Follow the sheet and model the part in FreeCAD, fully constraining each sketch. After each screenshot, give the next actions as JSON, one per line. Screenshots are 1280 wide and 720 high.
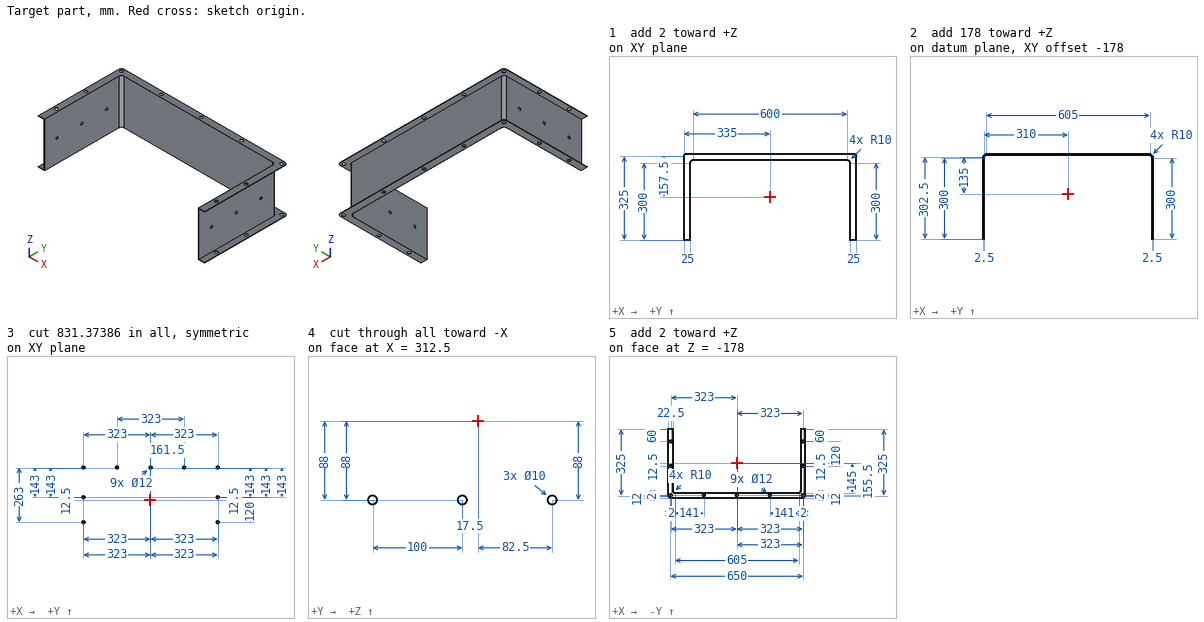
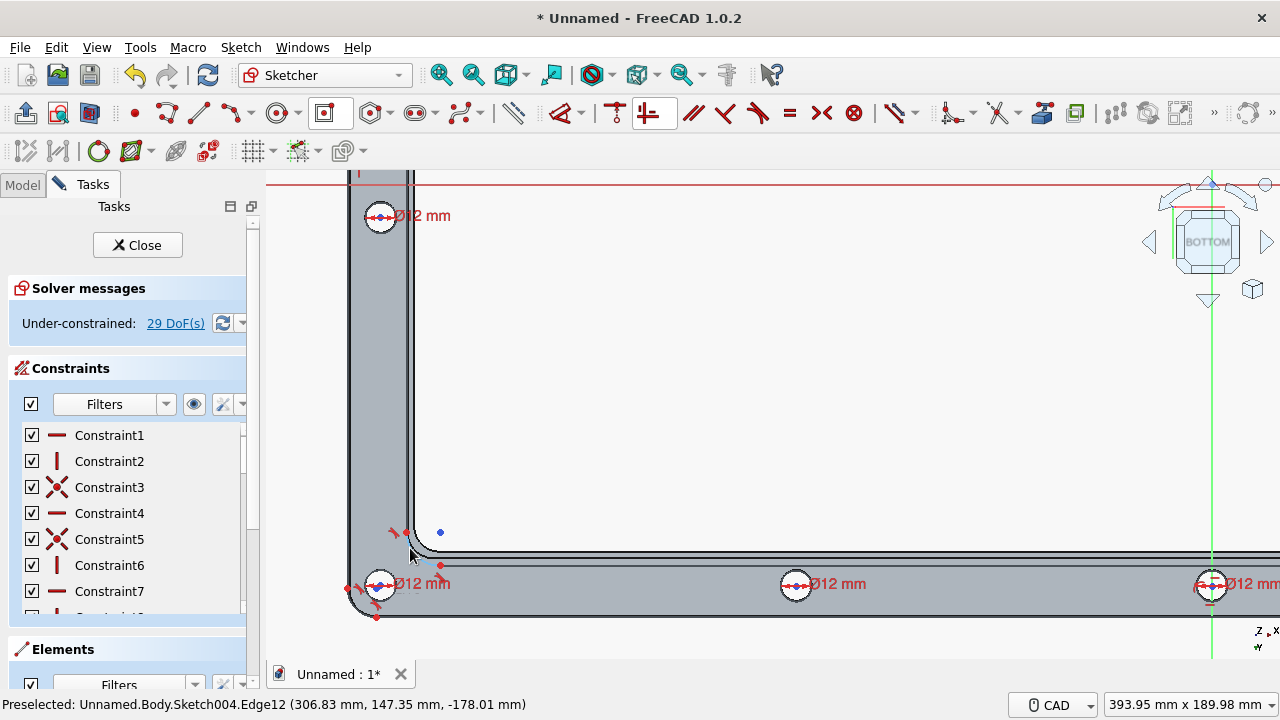
{"action": "left_click", "coordinate": [410, 547]}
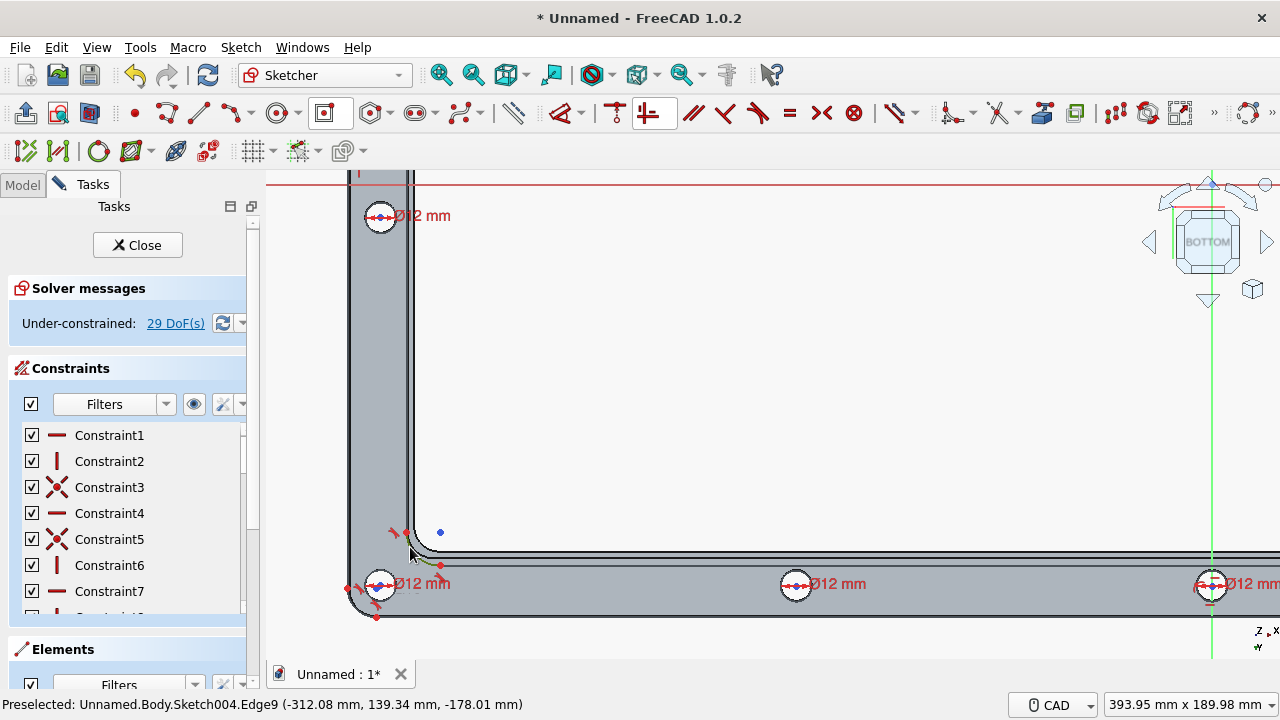
{"action": "left_click", "coordinate": [351, 602]}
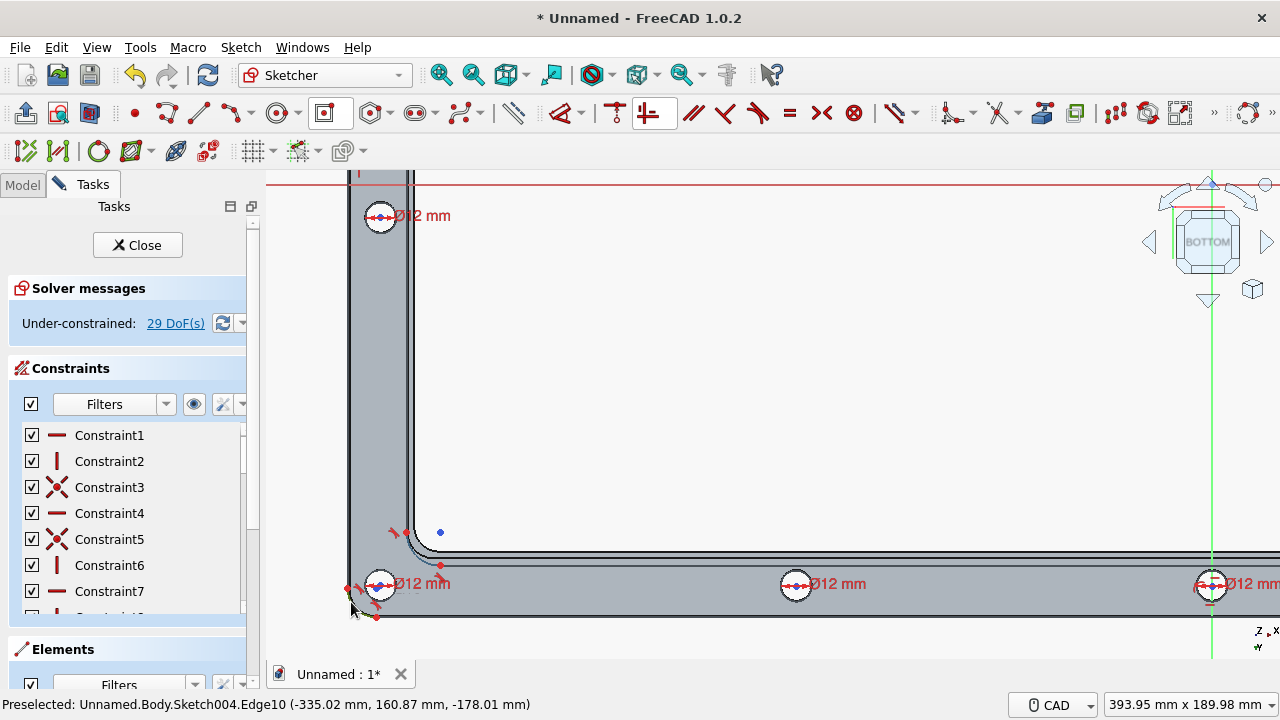
{"action": "scroll", "coordinate": [409, 548], "scroll_direction": "down", "scroll_amount": 5}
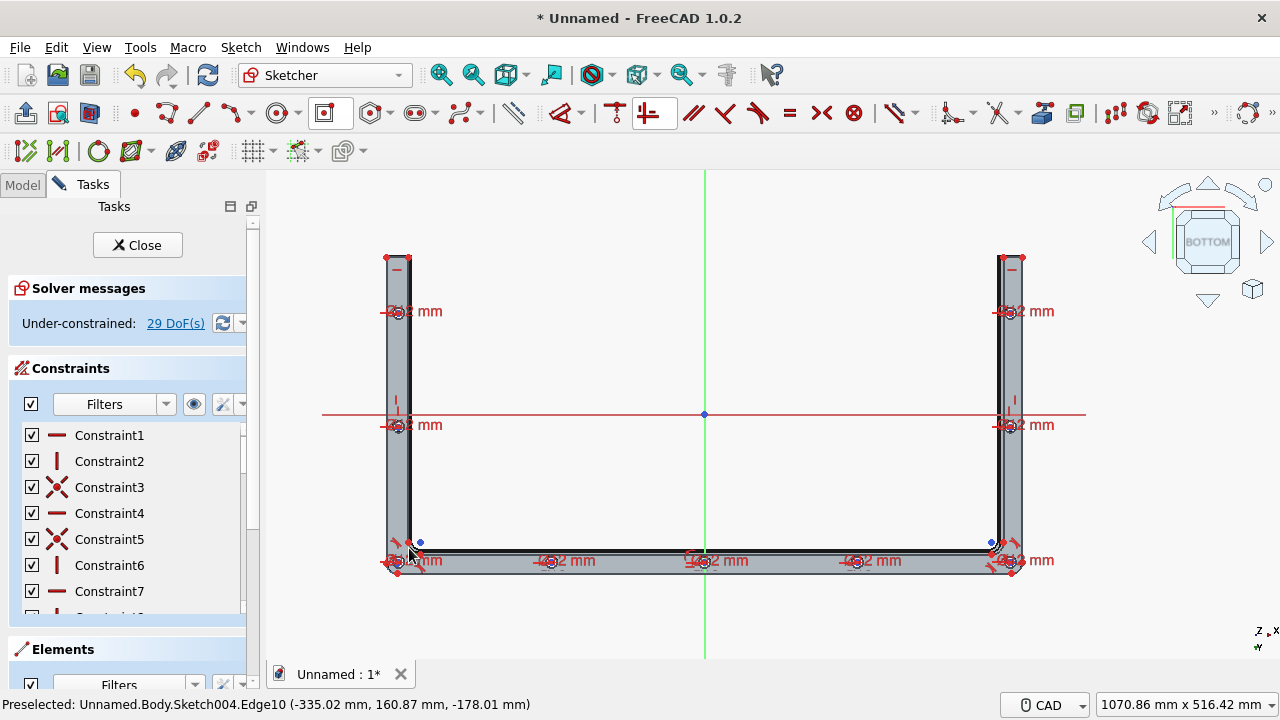
{"action": "scroll", "coordinate": [1016, 573], "scroll_direction": "up", "scroll_amount": 5}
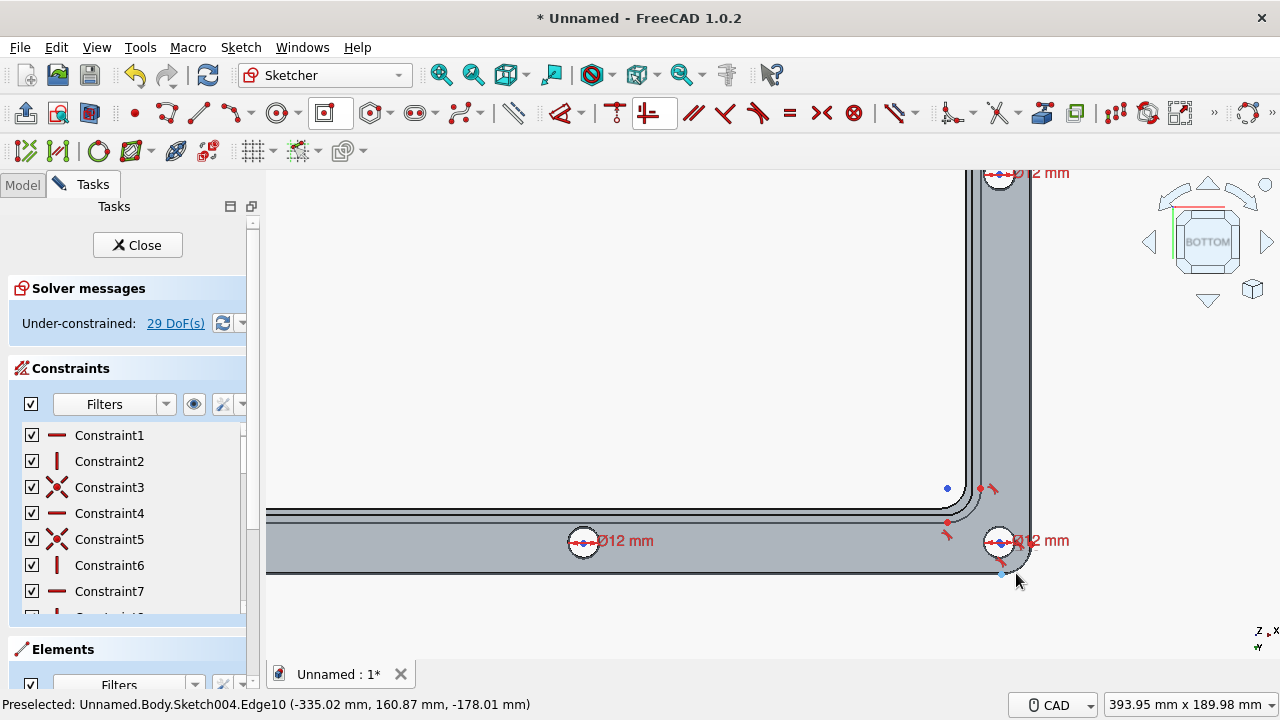
{"action": "left_click", "coordinate": [1015, 571]}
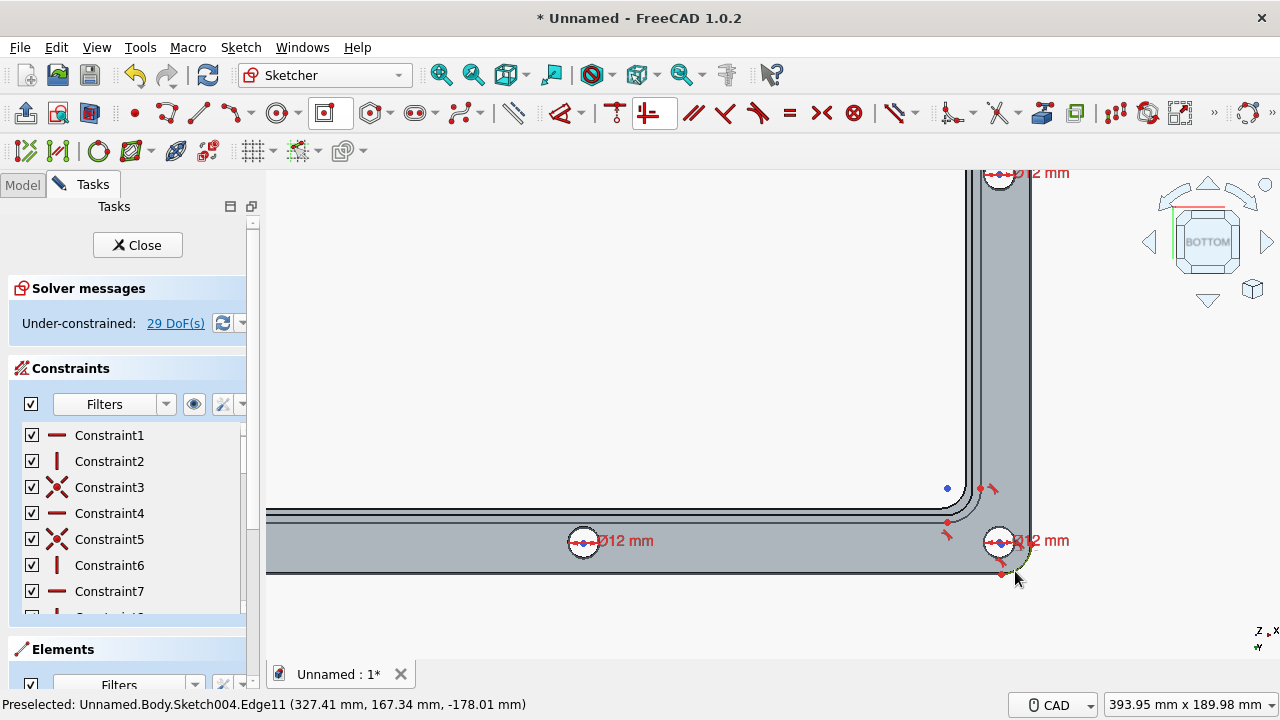
{"action": "left_click", "coordinate": [962, 519]}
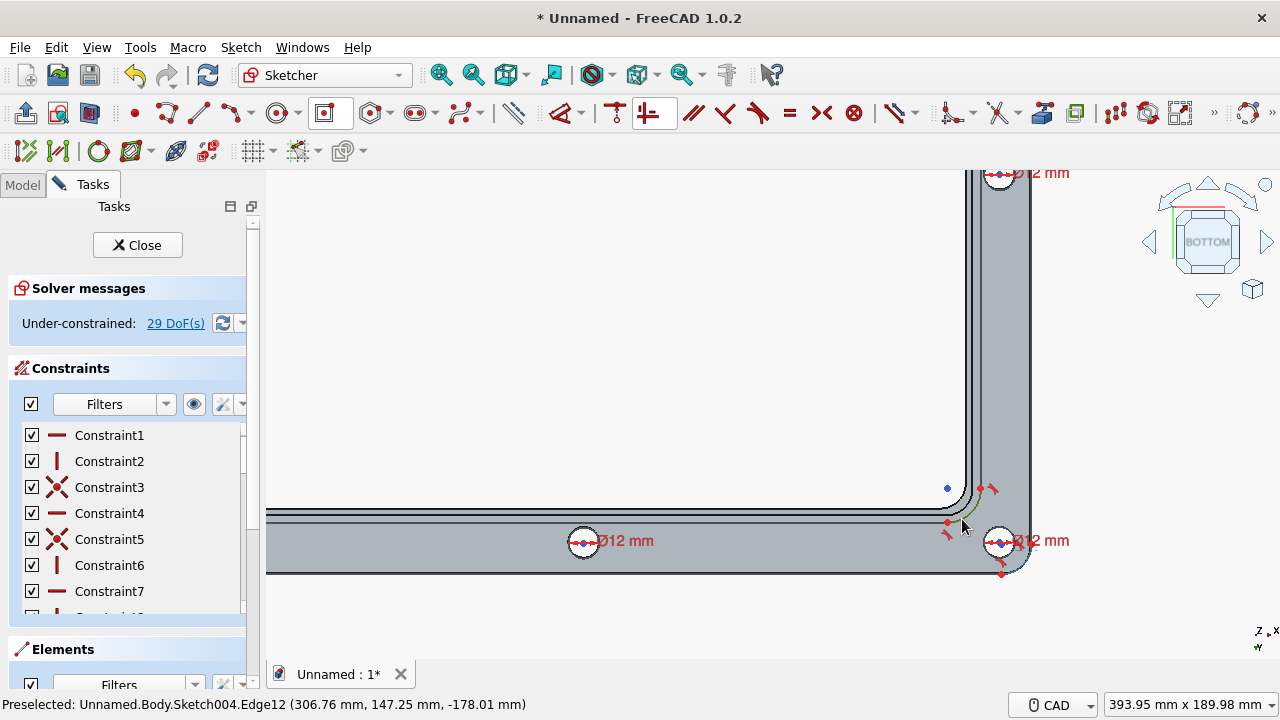
{"action": "left_click", "coordinate": [790, 114]}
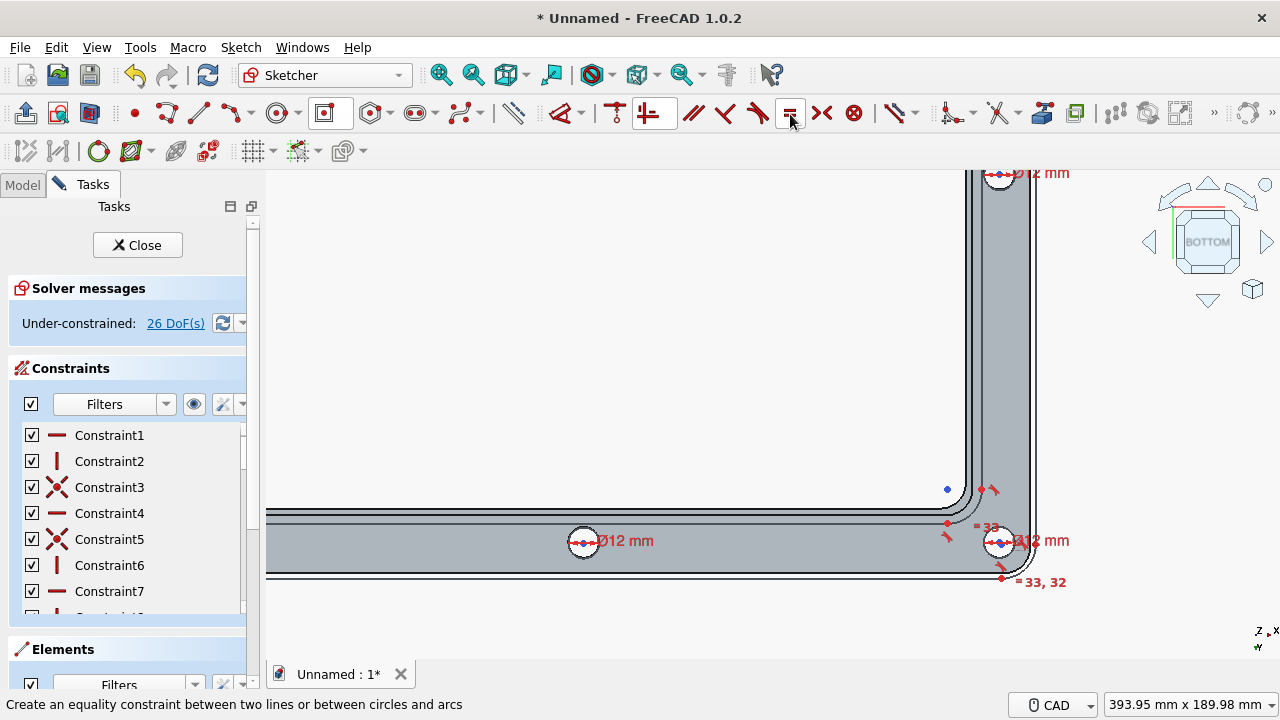
{"action": "left_click", "coordinate": [560, 114]}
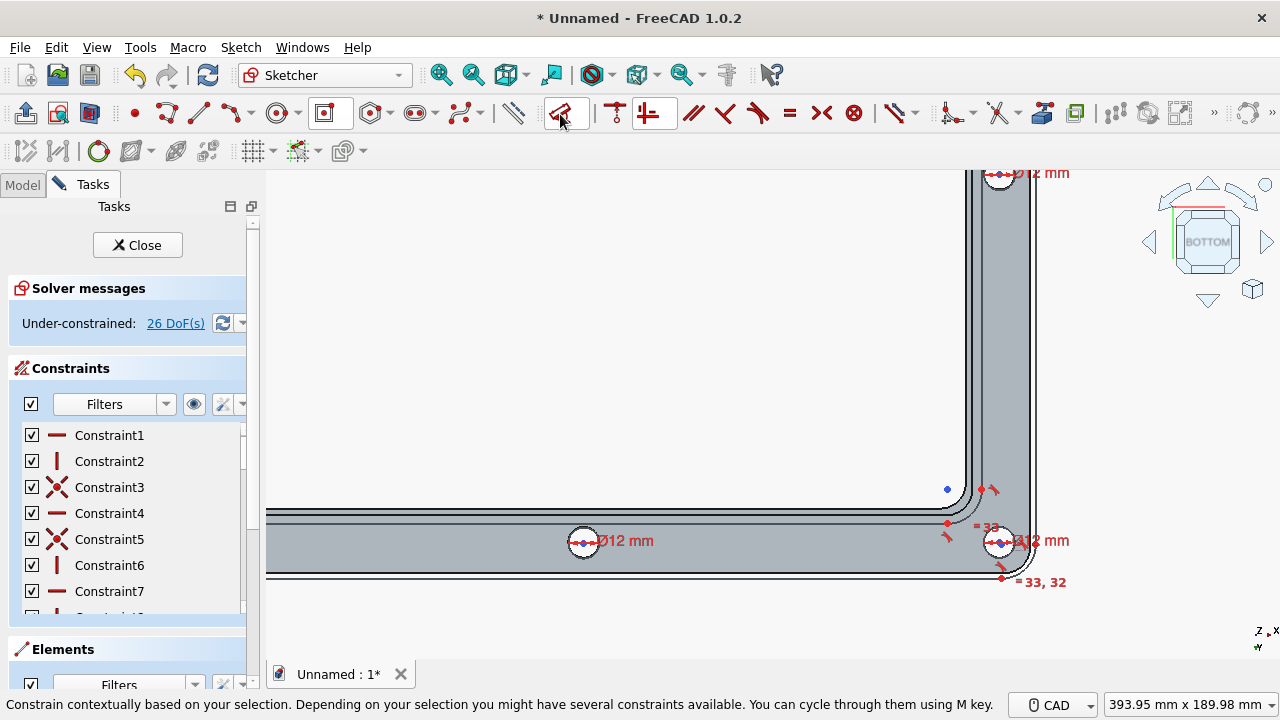
{"action": "scroll", "coordinate": [1017, 573], "scroll_direction": "down", "scroll_amount": 5}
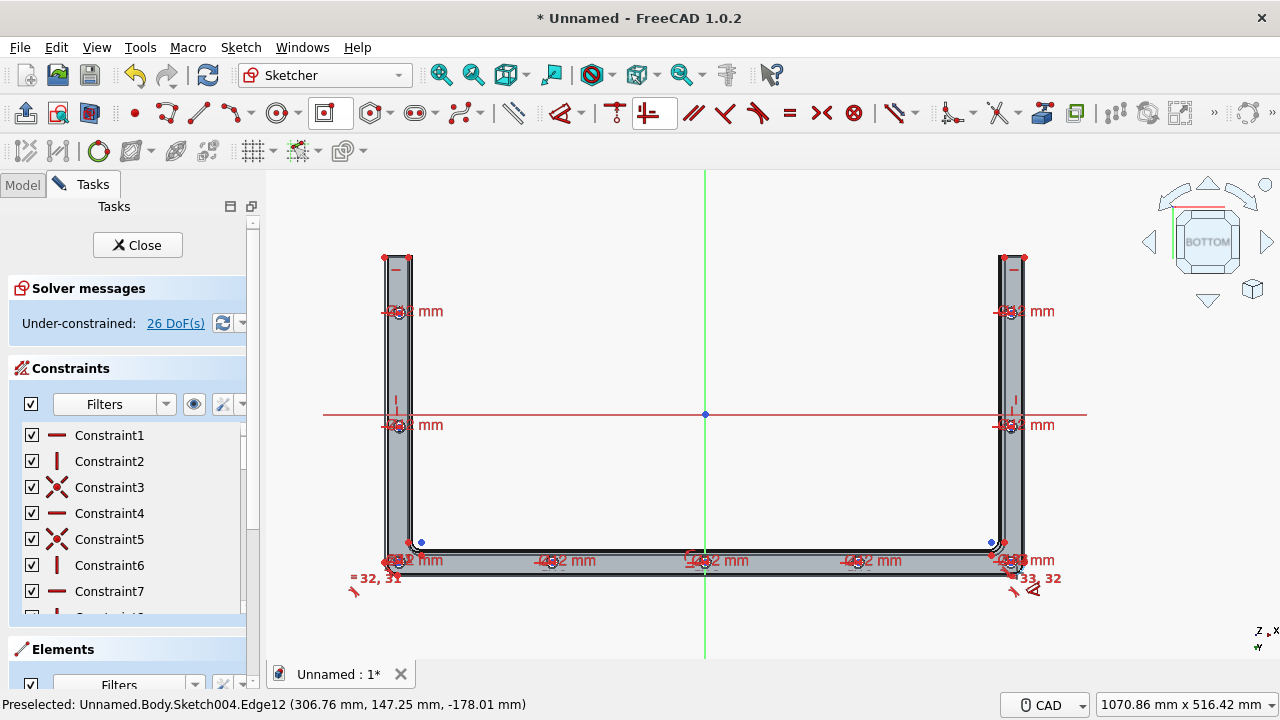
{"action": "scroll", "coordinate": [410, 548], "scroll_direction": "up", "scroll_amount": 8}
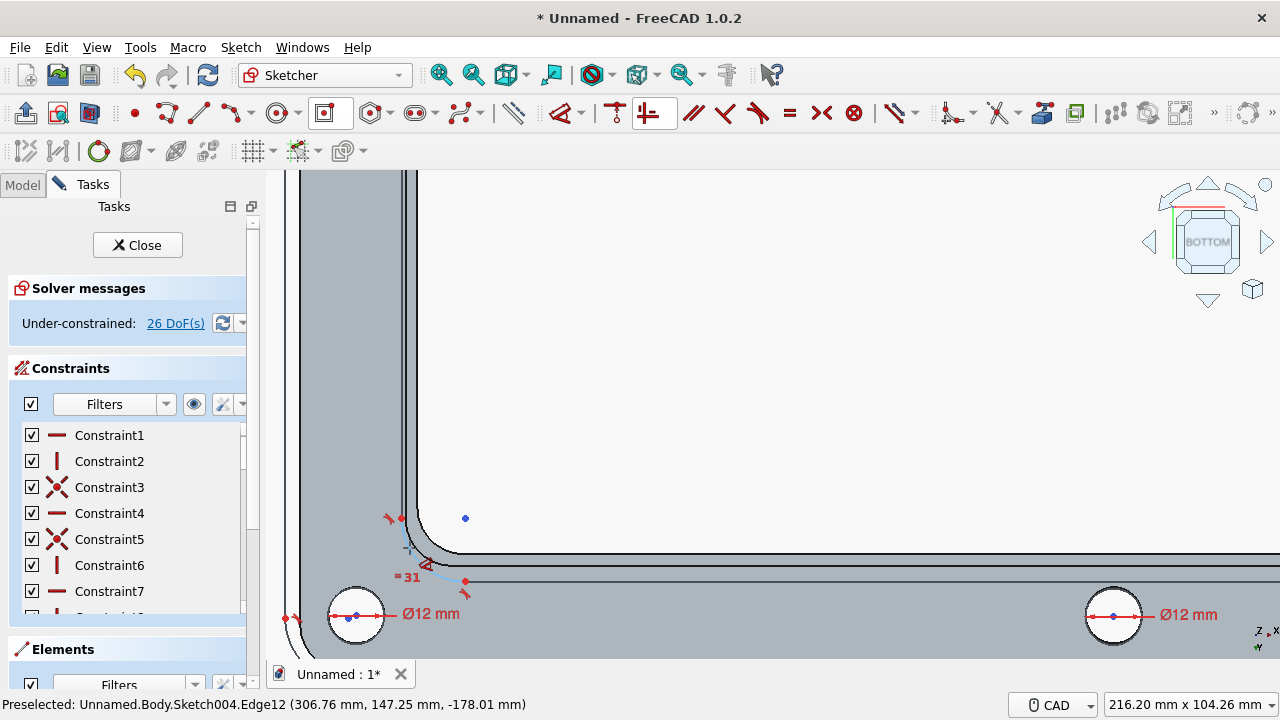
{"action": "left_click", "coordinate": [409, 547]}
{"action": "left_click", "coordinate": [380, 562]}